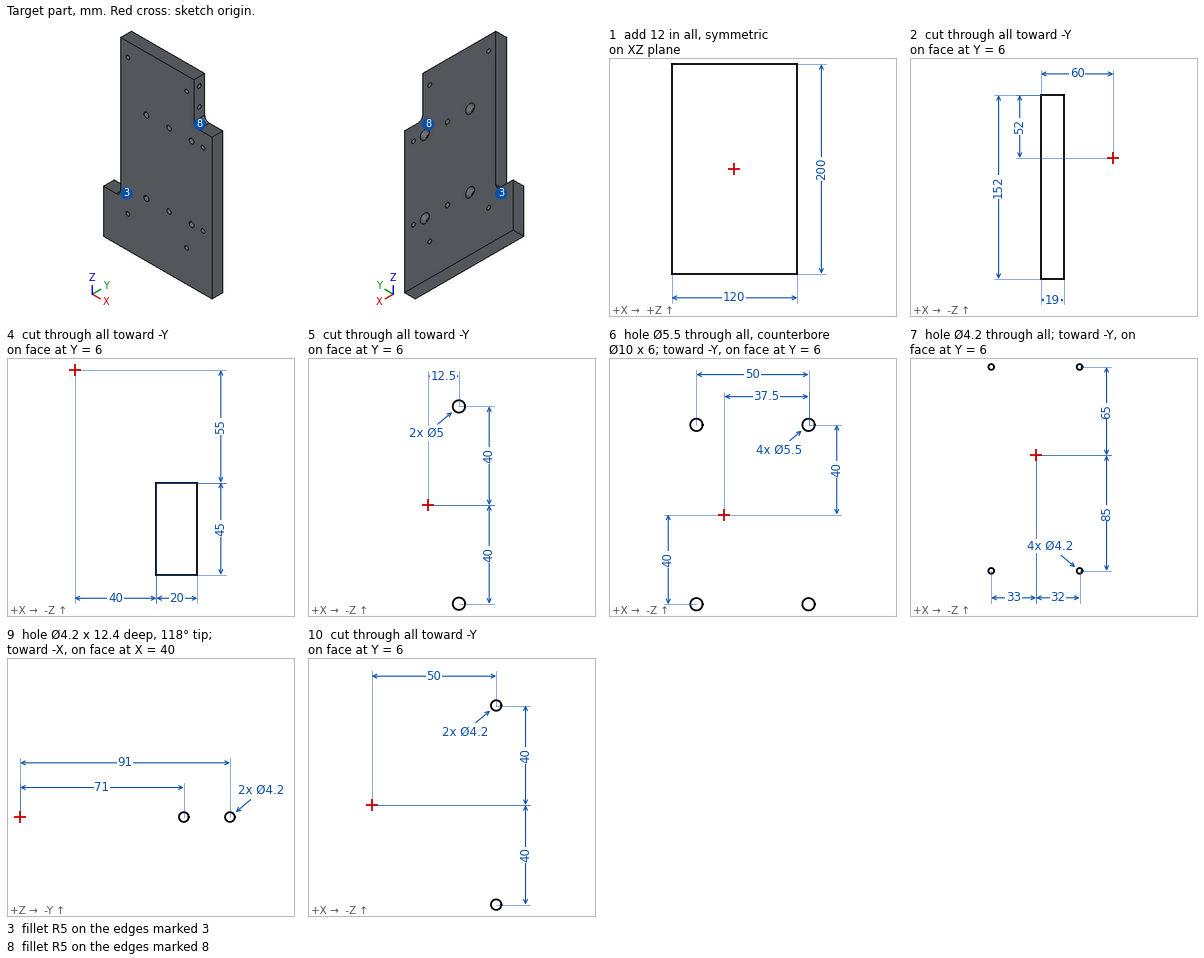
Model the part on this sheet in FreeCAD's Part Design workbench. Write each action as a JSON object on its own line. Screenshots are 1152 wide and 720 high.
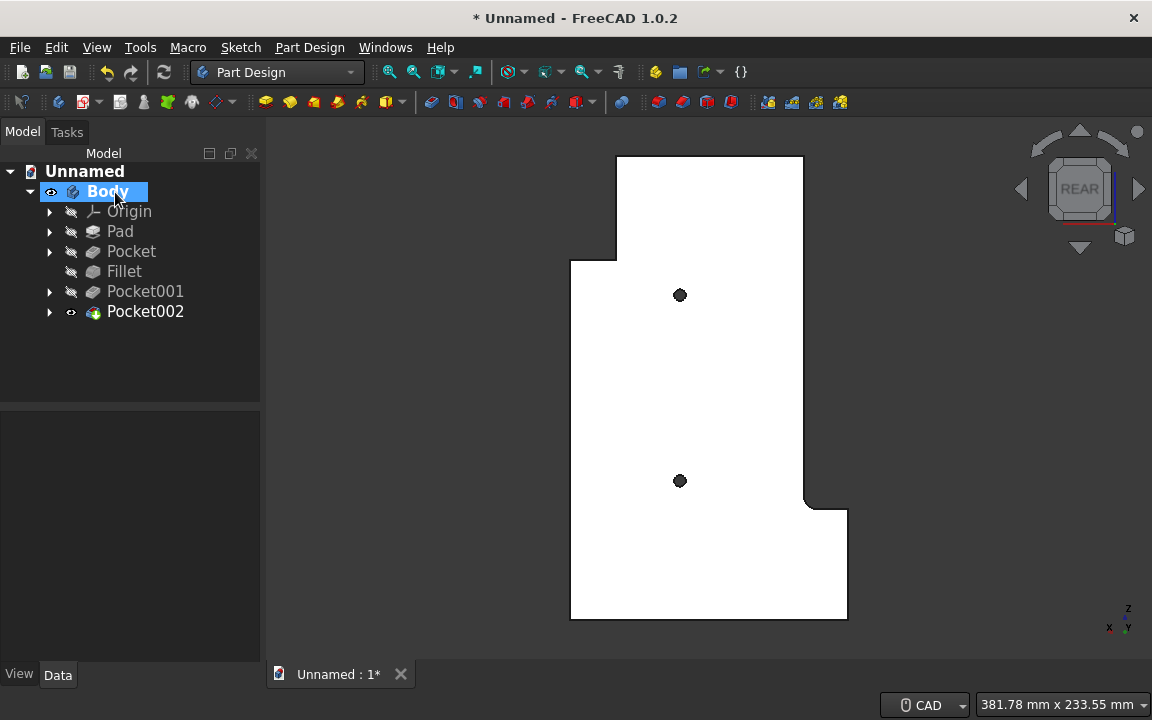
{"action": "left_click", "coordinate": [709, 387]}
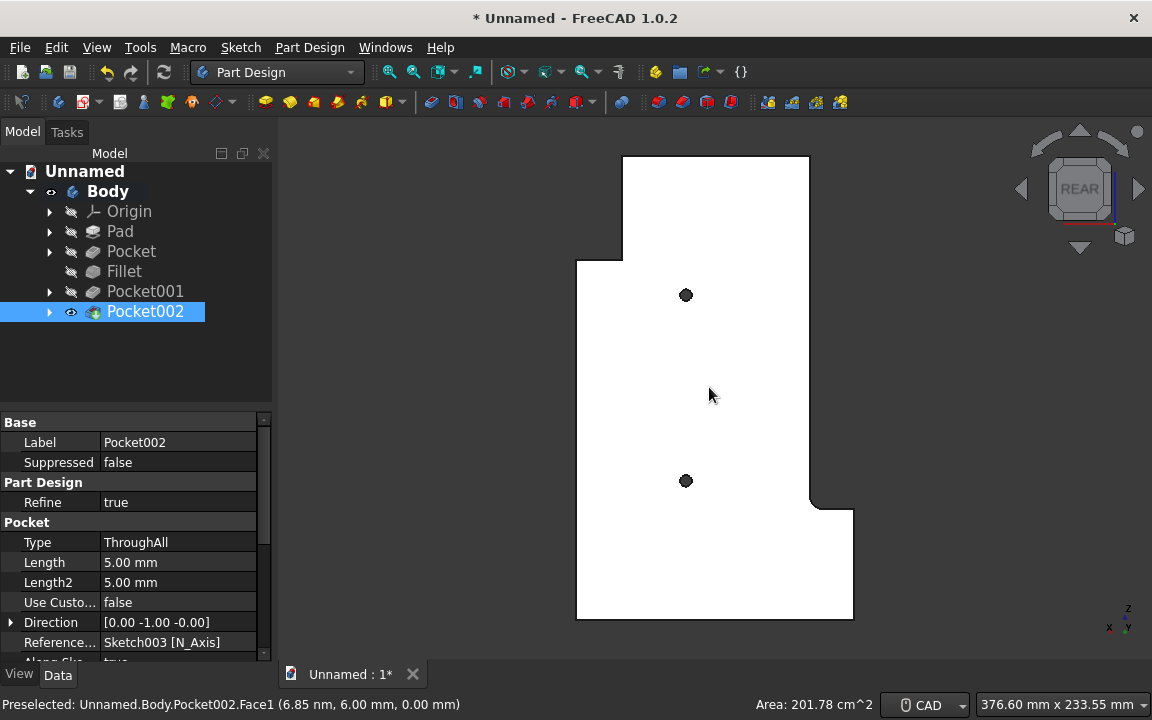
{"action": "left_click", "coordinate": [84, 102]}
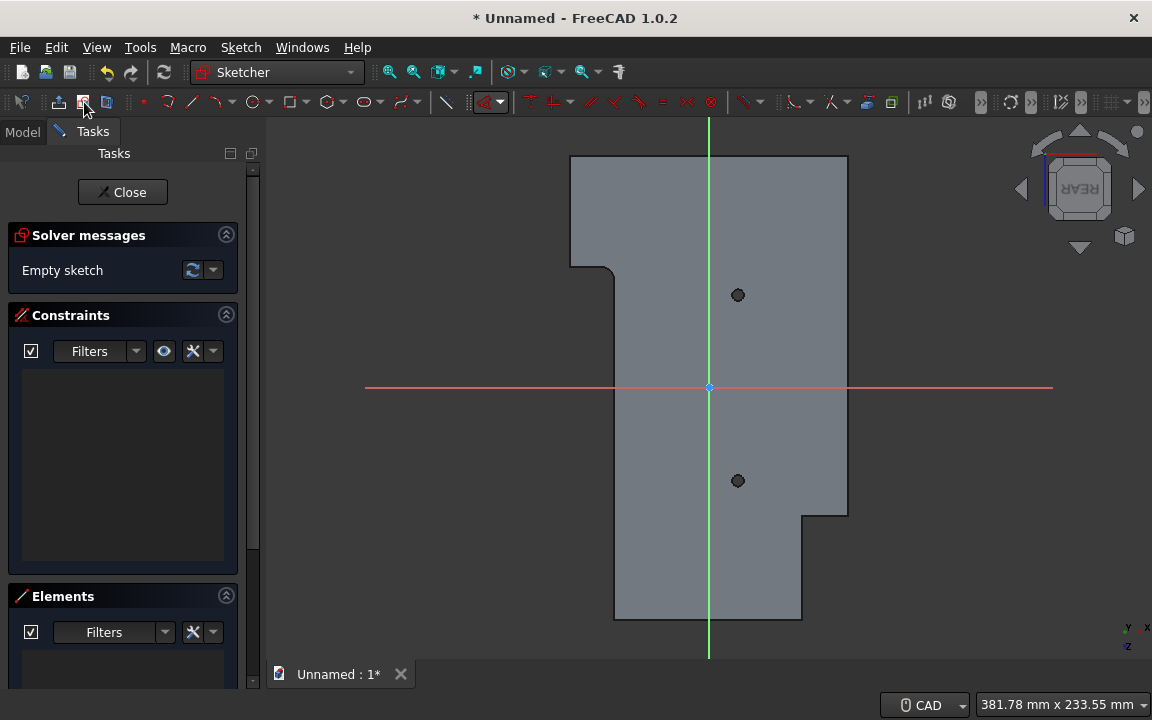
{"action": "scroll", "coordinate": [857, 388], "scroll_direction": "up", "scroll_amount": 3}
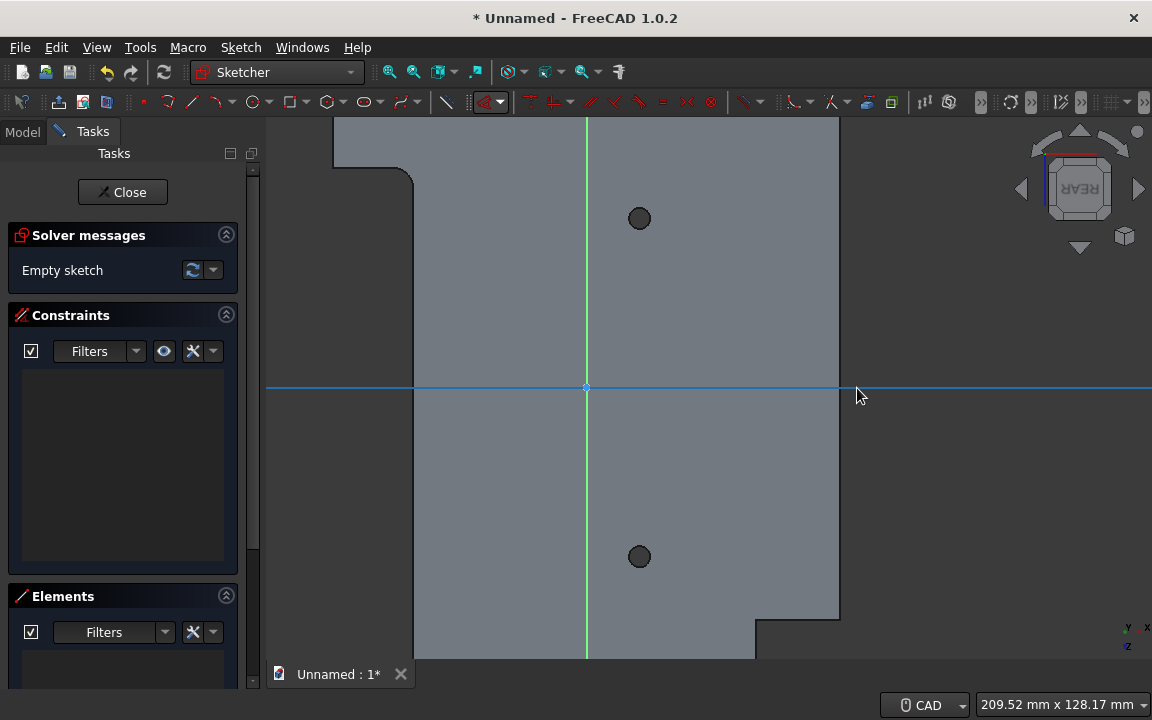
{"action": "left_click", "coordinate": [254, 102]}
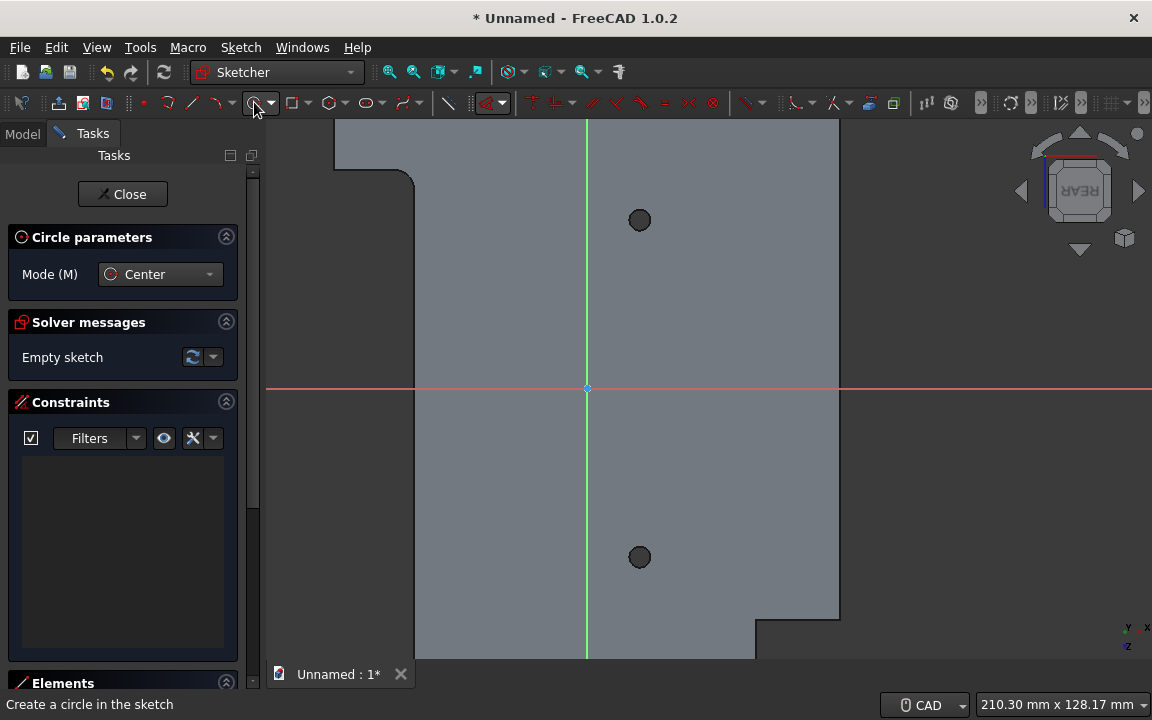
{"action": "scroll", "coordinate": [745, 220], "scroll_direction": "up", "scroll_amount": 4}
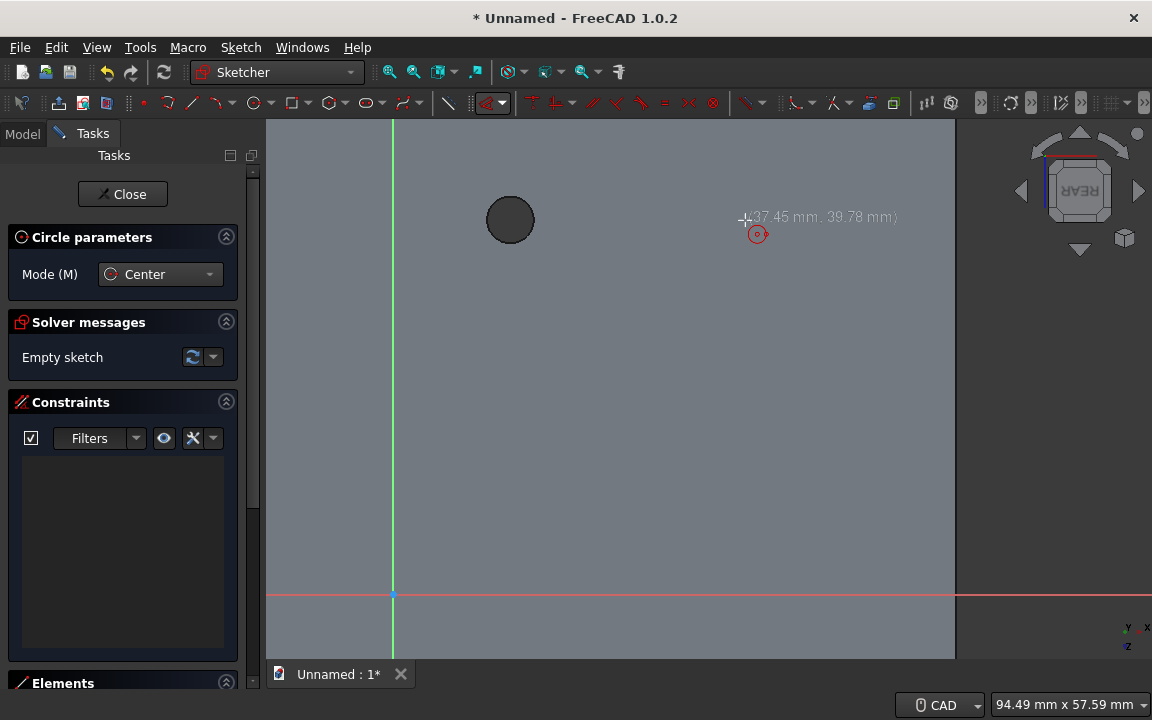
{"action": "left_click", "coordinate": [745, 220]}
{"action": "left_click", "coordinate": [763, 202]}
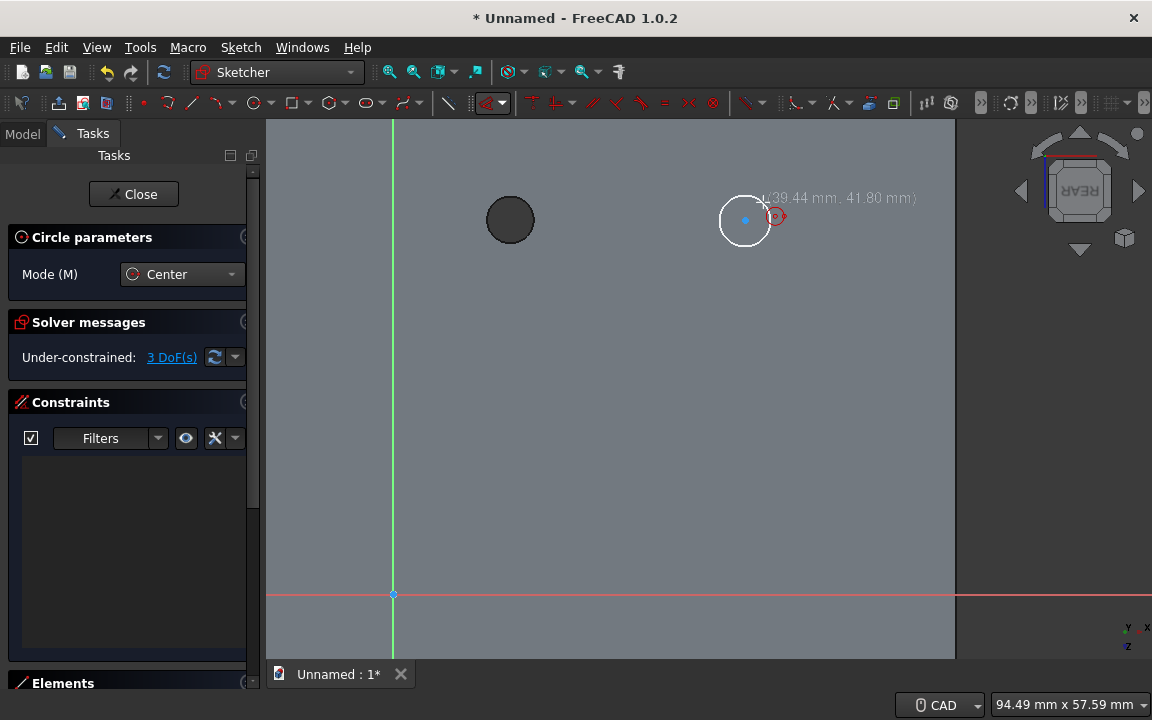
{"action": "scroll", "coordinate": [747, 221], "scroll_direction": "down", "scroll_amount": 4}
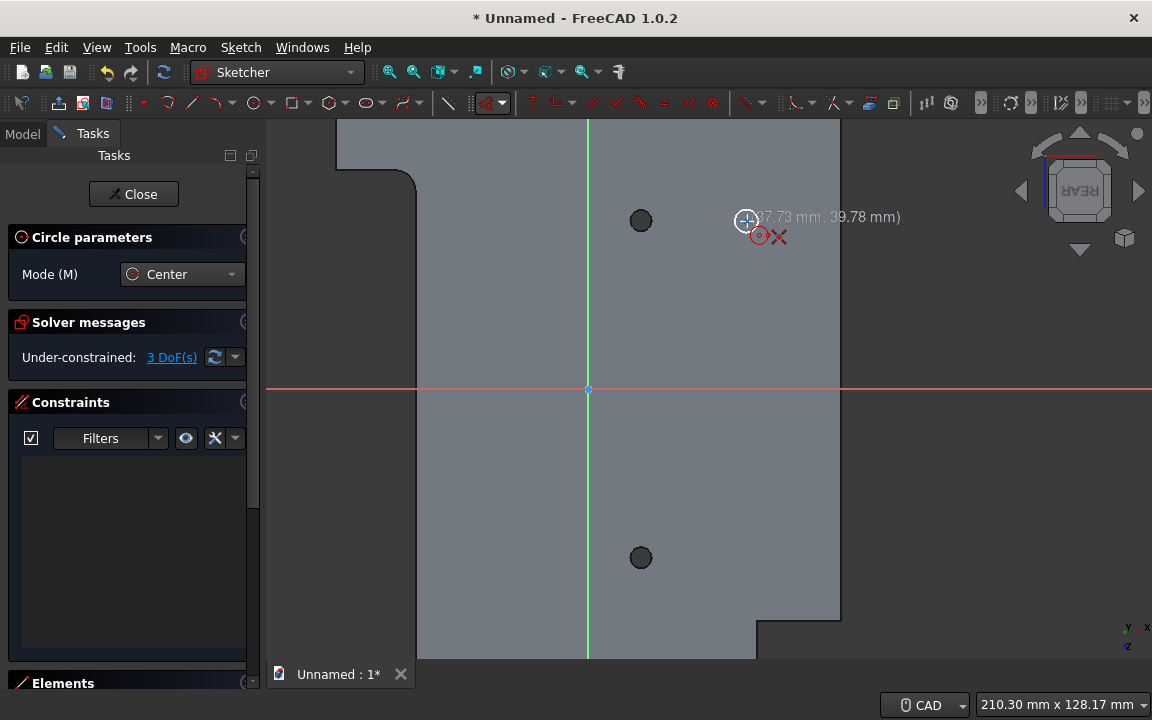
{"action": "scroll", "coordinate": [536, 221], "scroll_direction": "up", "scroll_amount": 4}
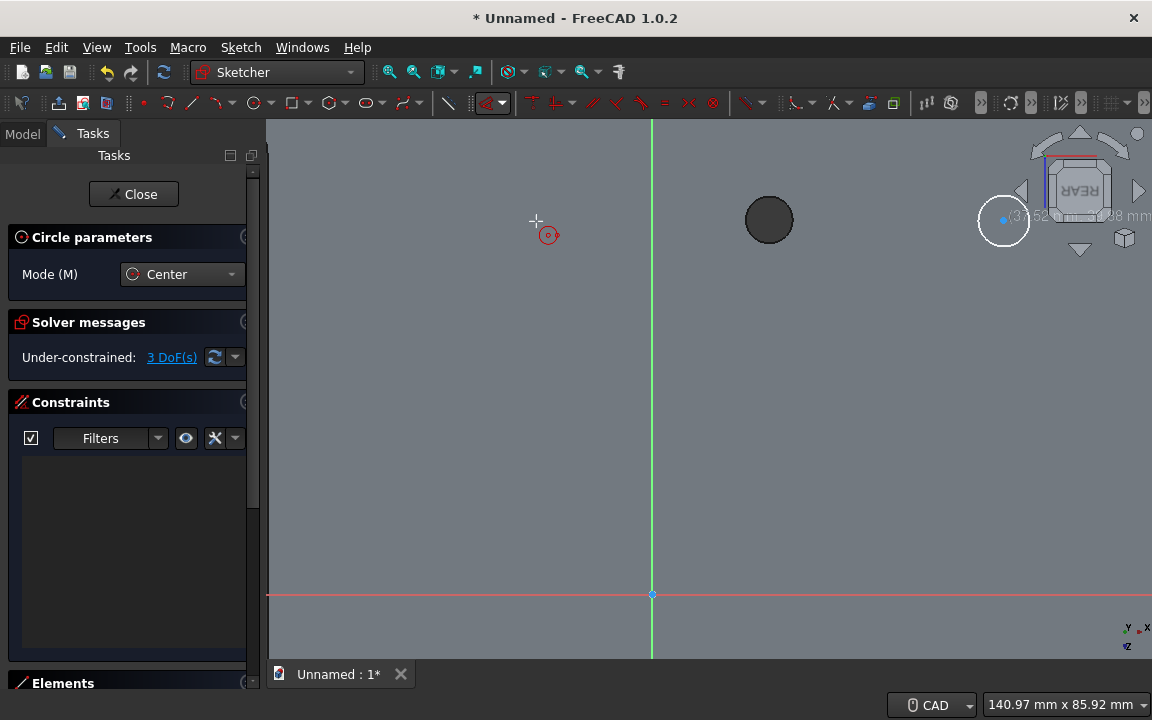
{"action": "left_click", "coordinate": [535, 220]}
{"action": "left_click", "coordinate": [553, 202]}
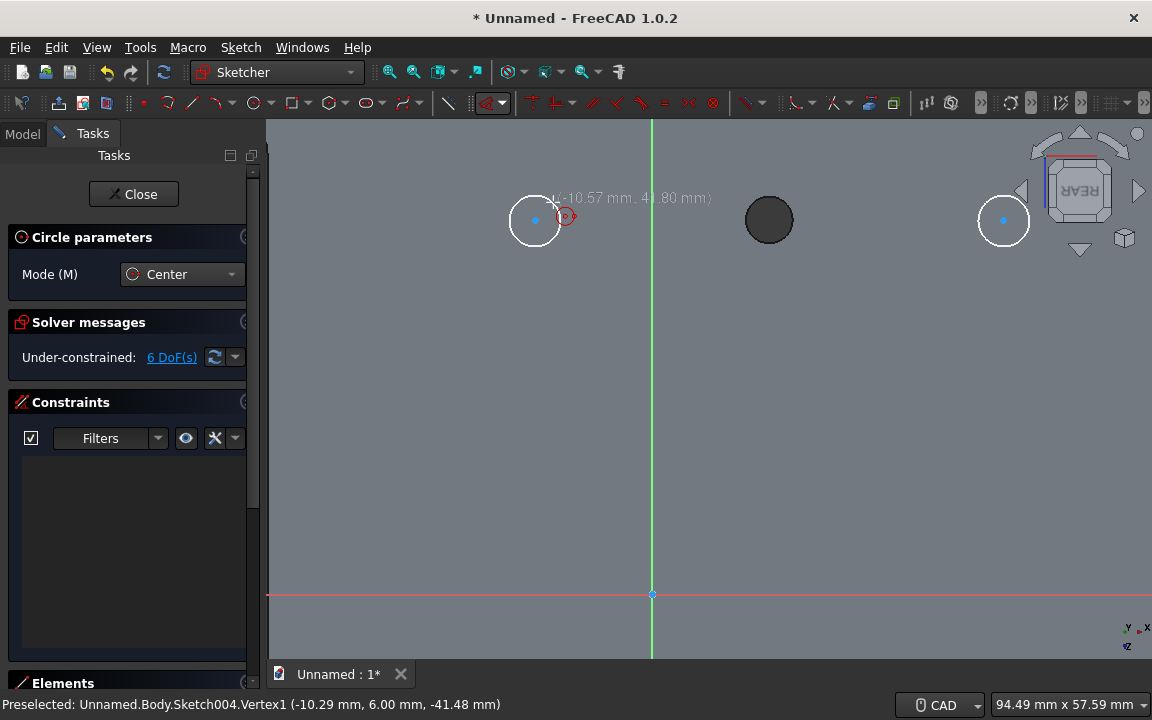
{"action": "scroll", "coordinate": [535, 221], "scroll_direction": "down", "scroll_amount": 4}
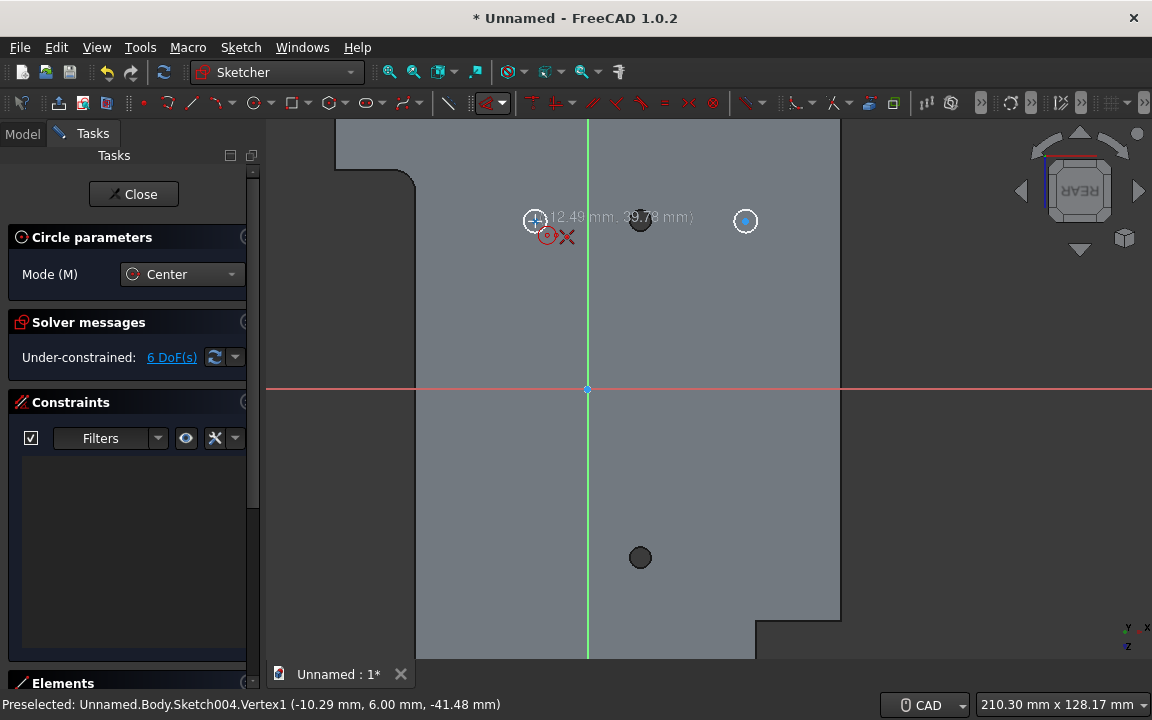
{"action": "scroll", "coordinate": [535, 558], "scroll_direction": "up", "scroll_amount": 4}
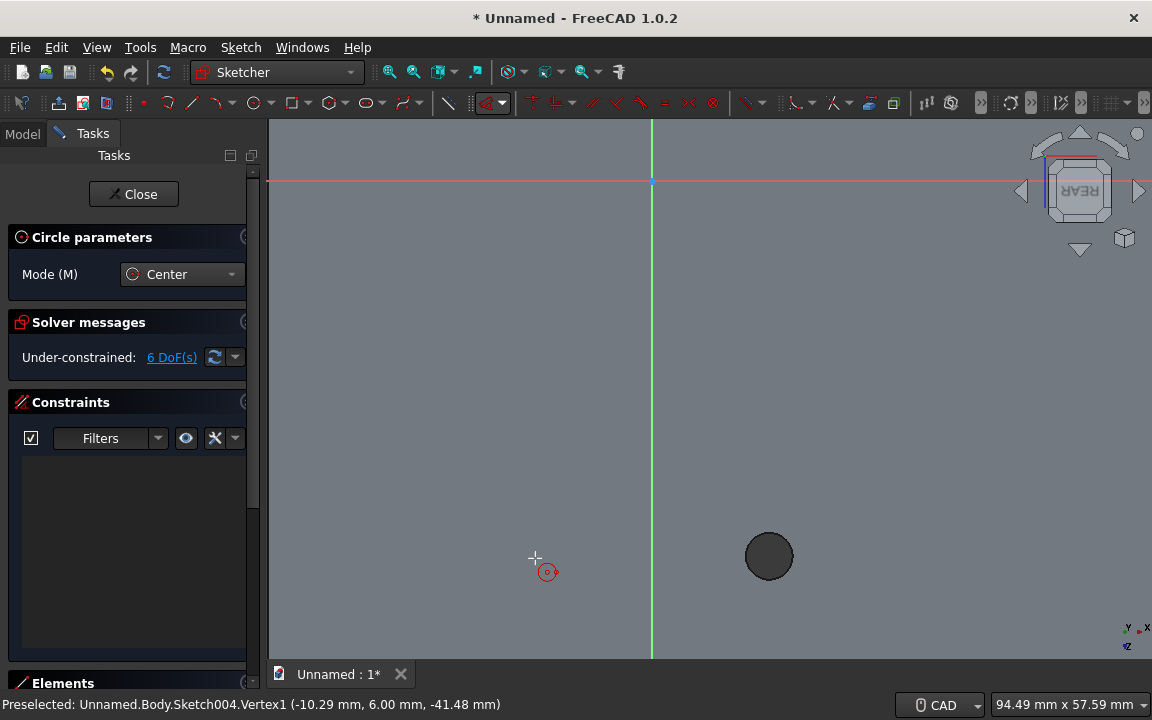
{"action": "left_click", "coordinate": [535, 556]}
{"action": "left_click", "coordinate": [553, 538]}